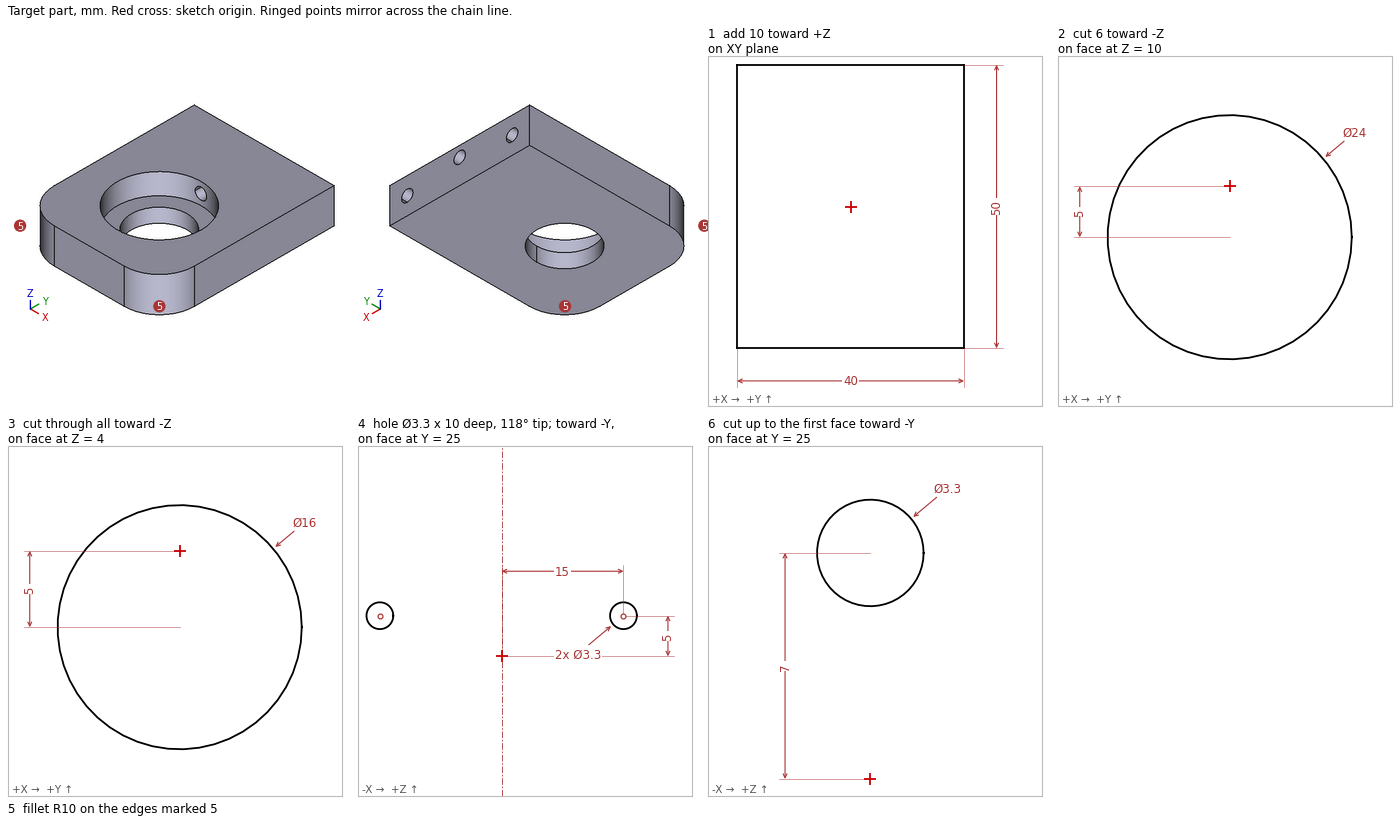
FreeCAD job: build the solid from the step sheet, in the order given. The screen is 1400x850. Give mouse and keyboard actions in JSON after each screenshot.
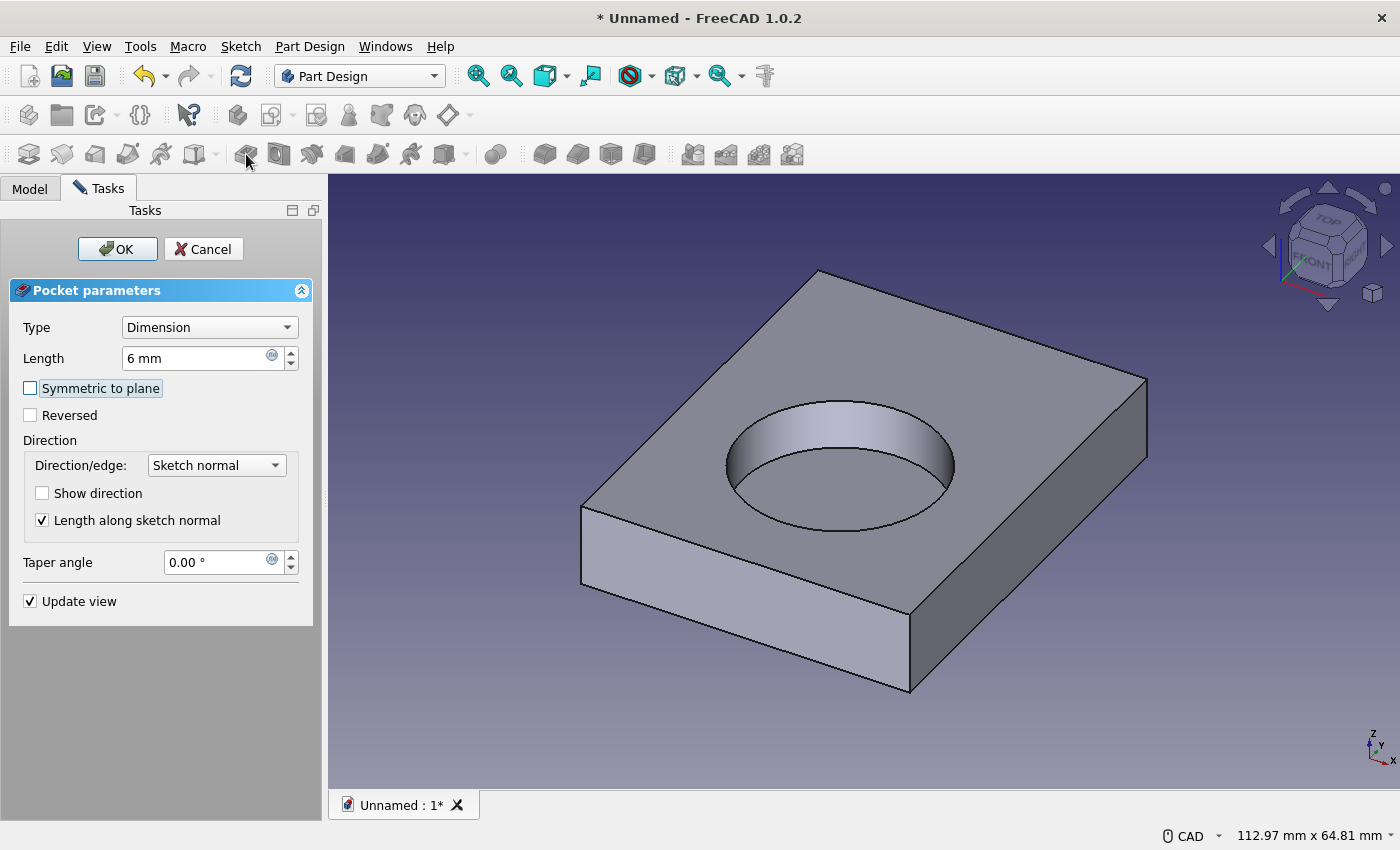
{"action": "left_click", "coordinate": [118, 249]}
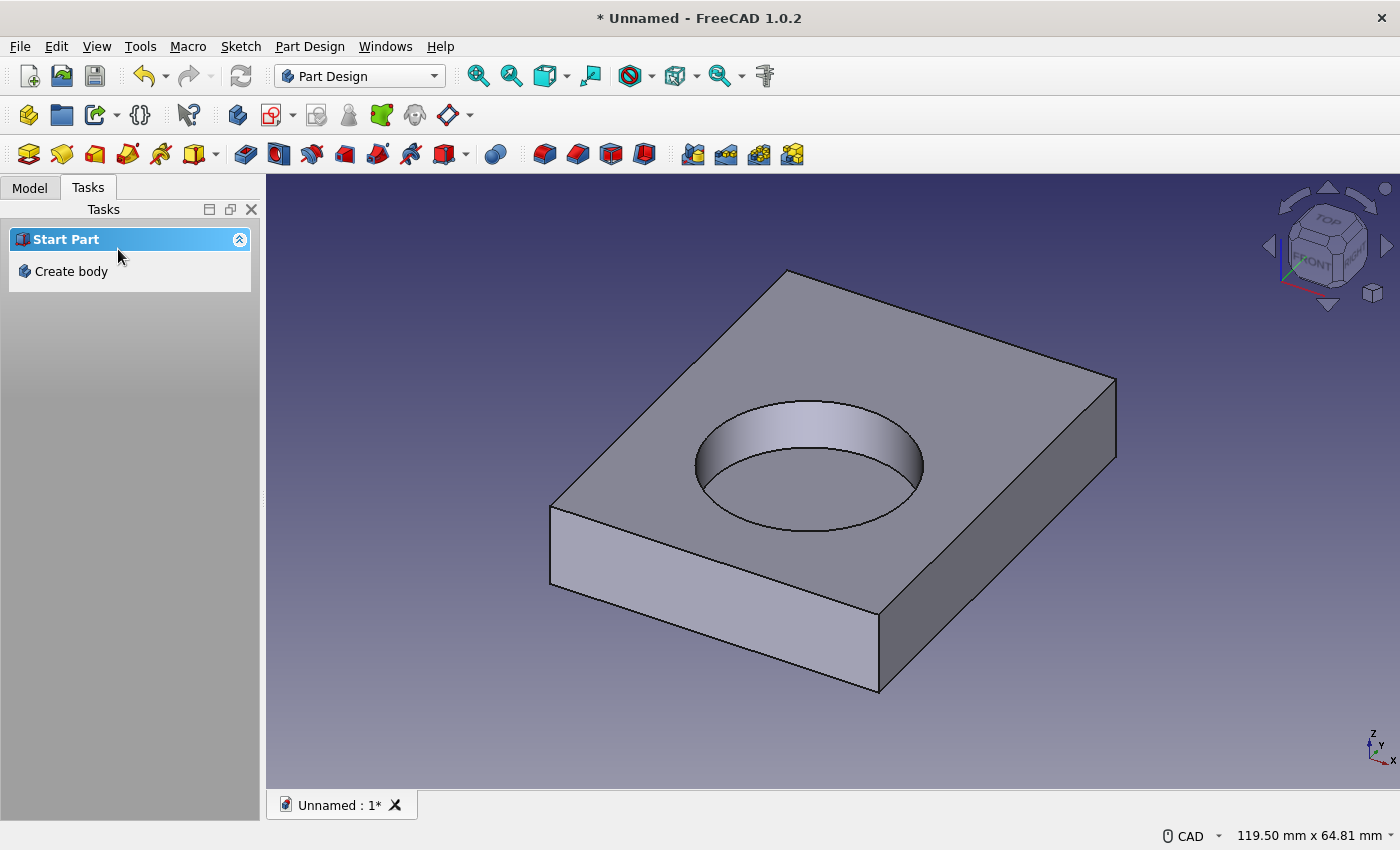
{"action": "left_click", "coordinate": [809, 512]}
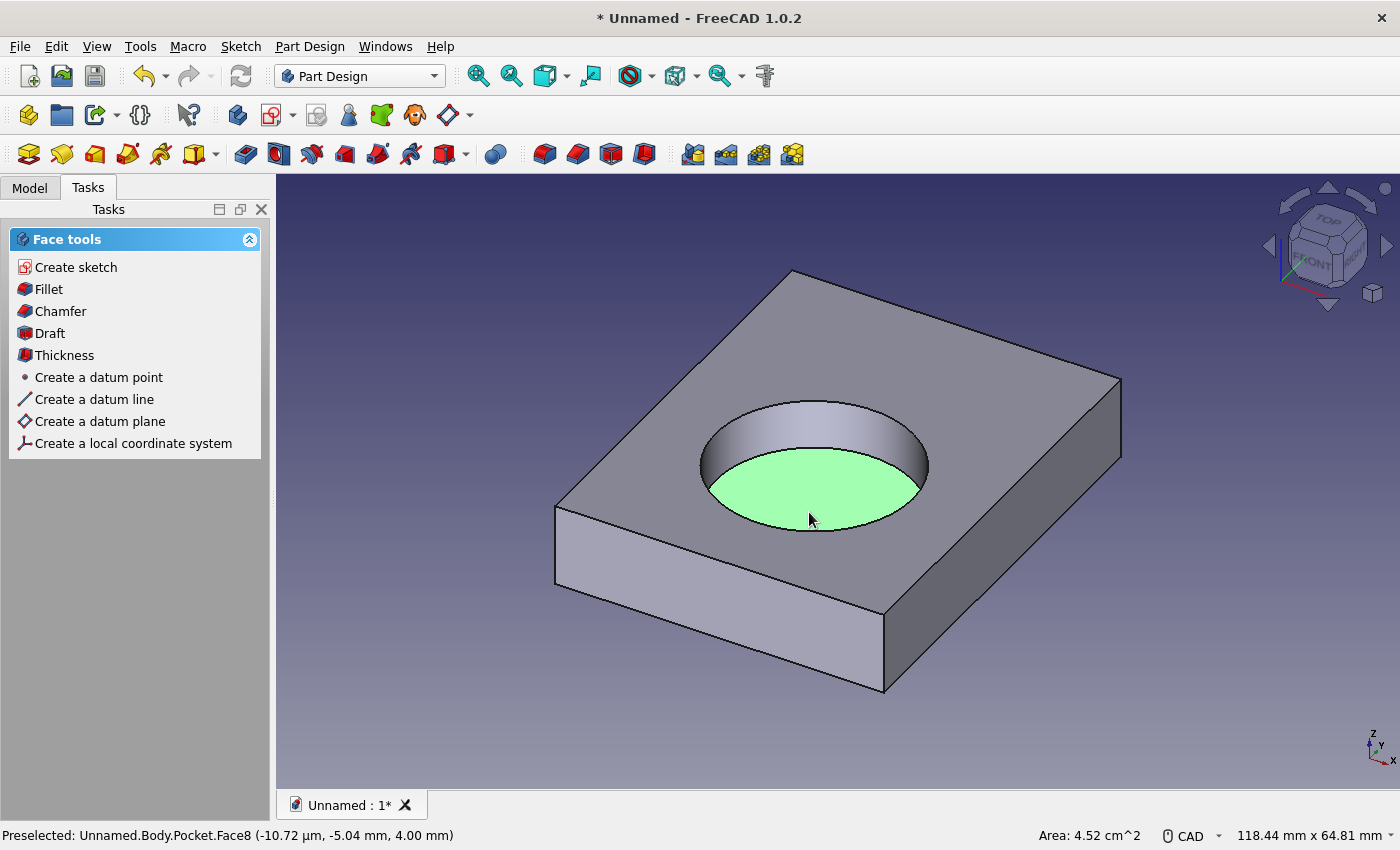
{"action": "left_click", "coordinate": [270, 116]}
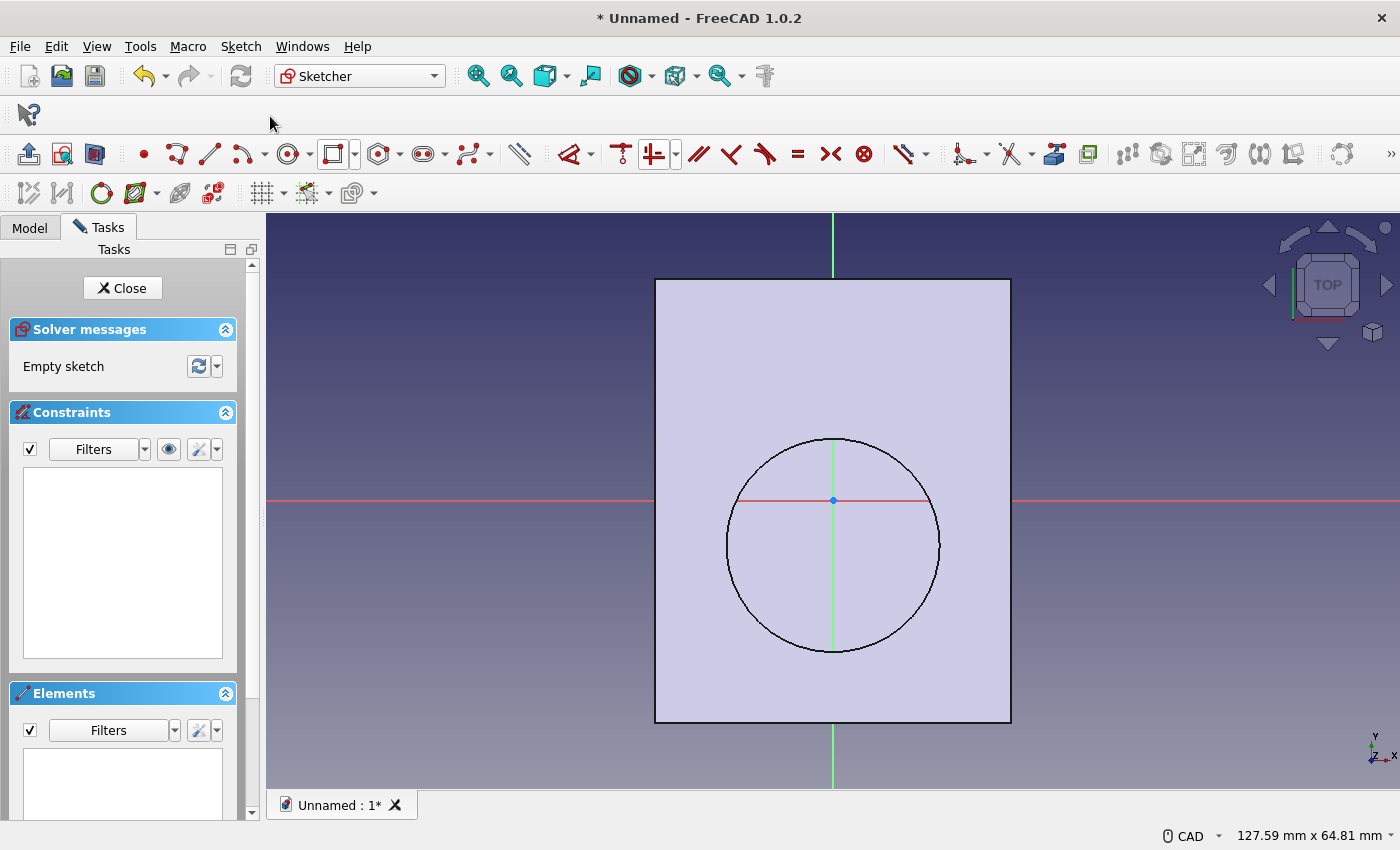
{"action": "left_click", "coordinate": [95, 154]}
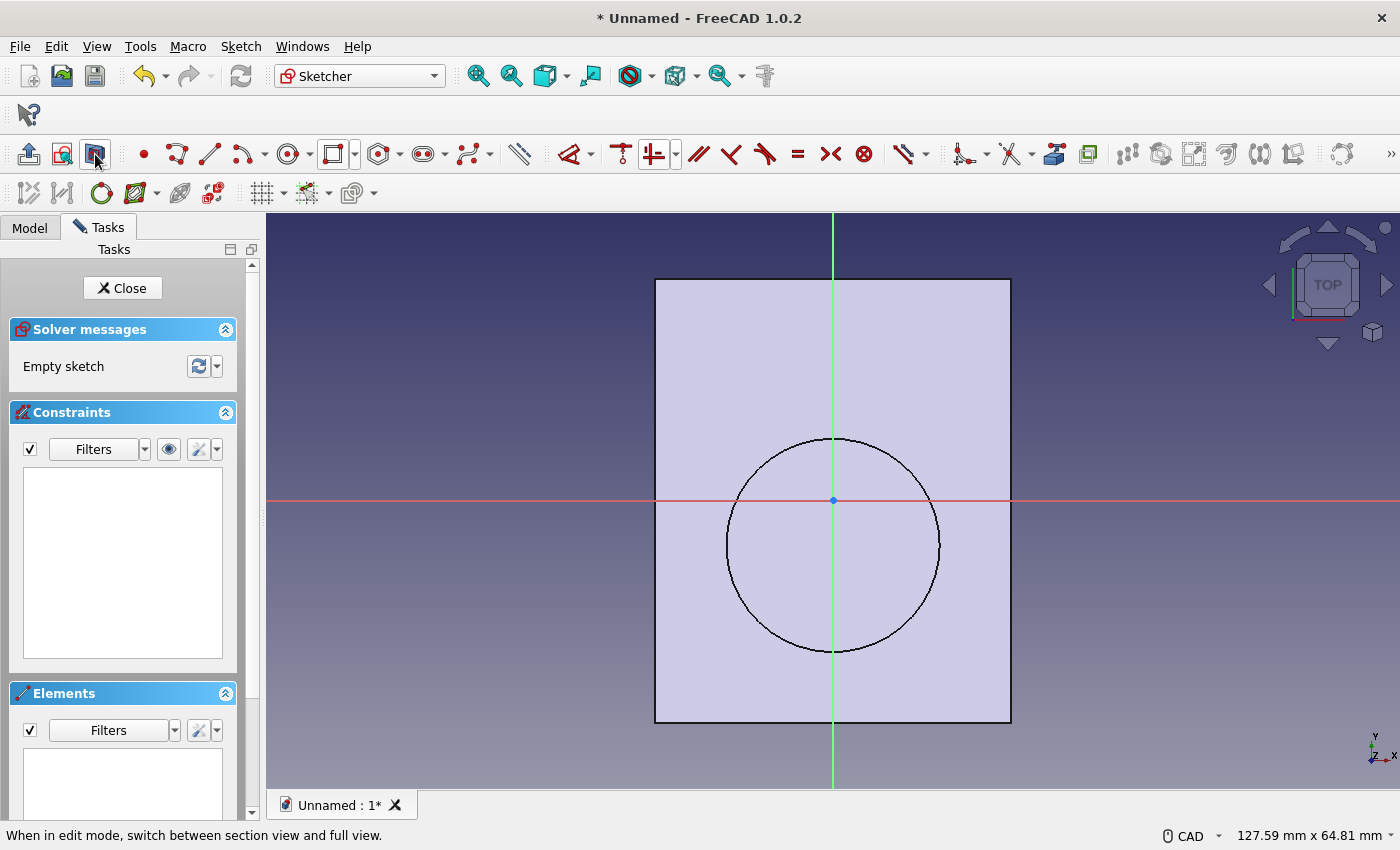
{"action": "scroll", "coordinate": [873, 571], "scroll_direction": "up", "scroll_amount": 5}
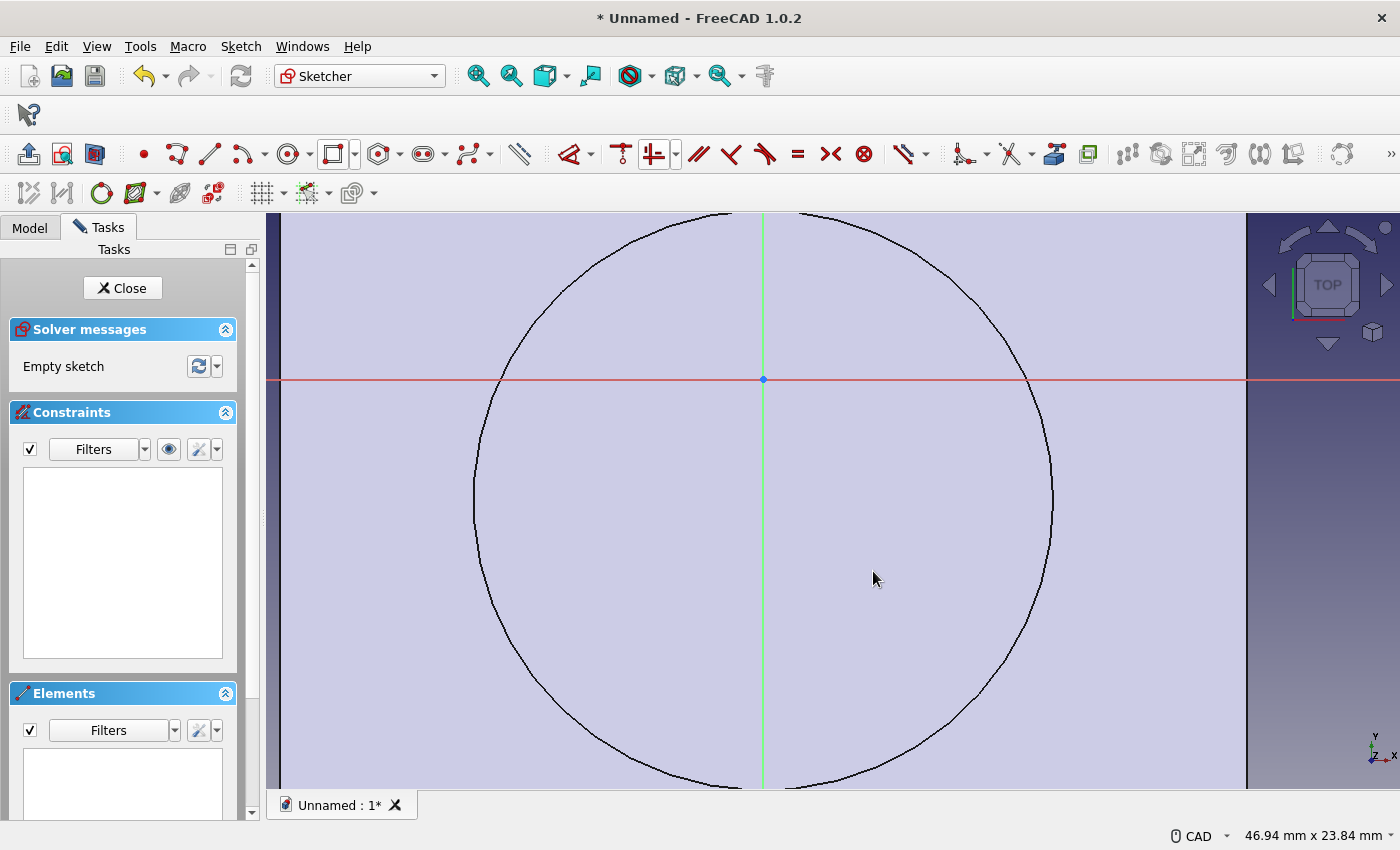
{"action": "left_click", "coordinate": [288, 154]}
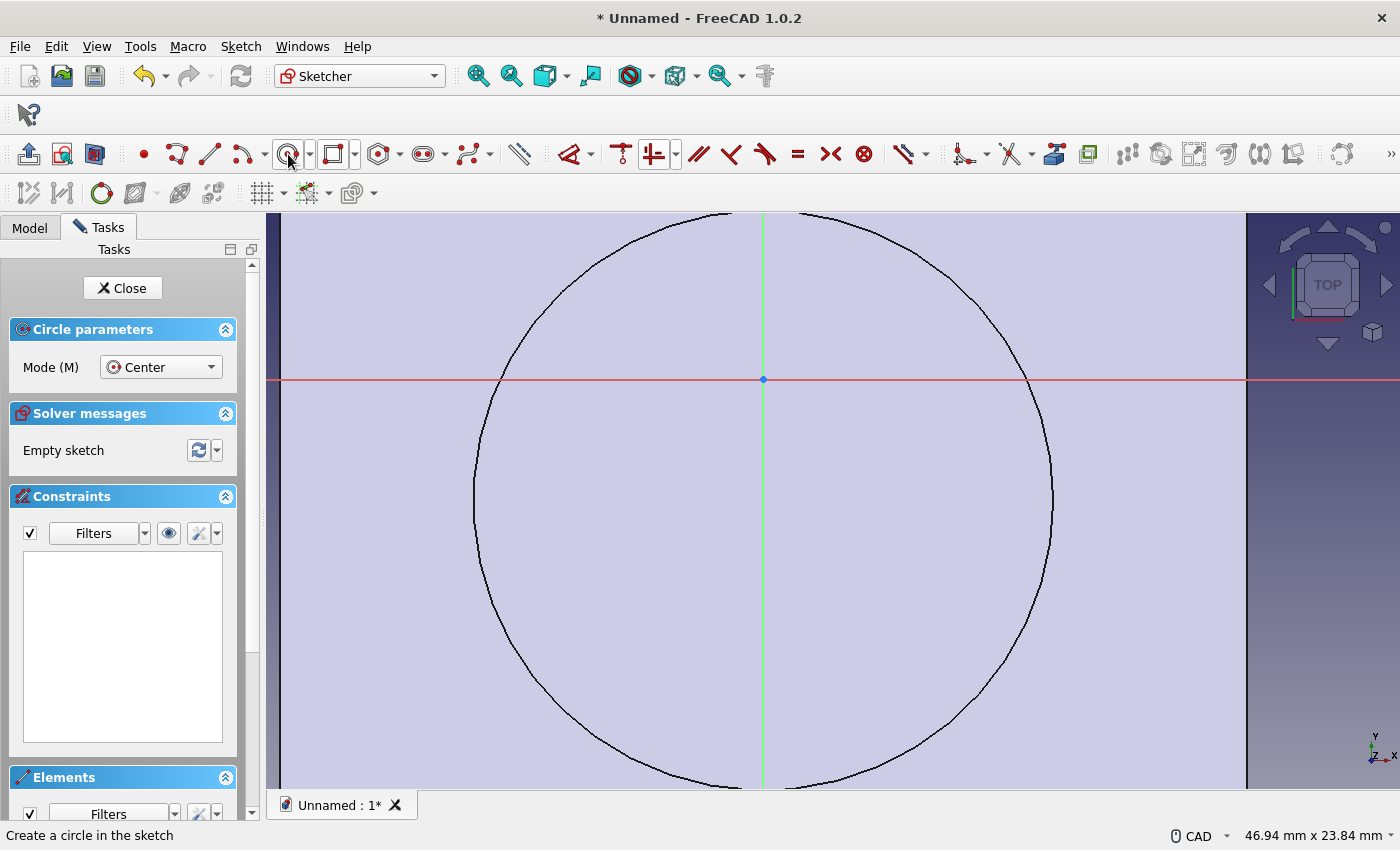
{"action": "left_click", "coordinate": [763, 500]}
{"action": "mouse_move", "coordinate": [900, 364]}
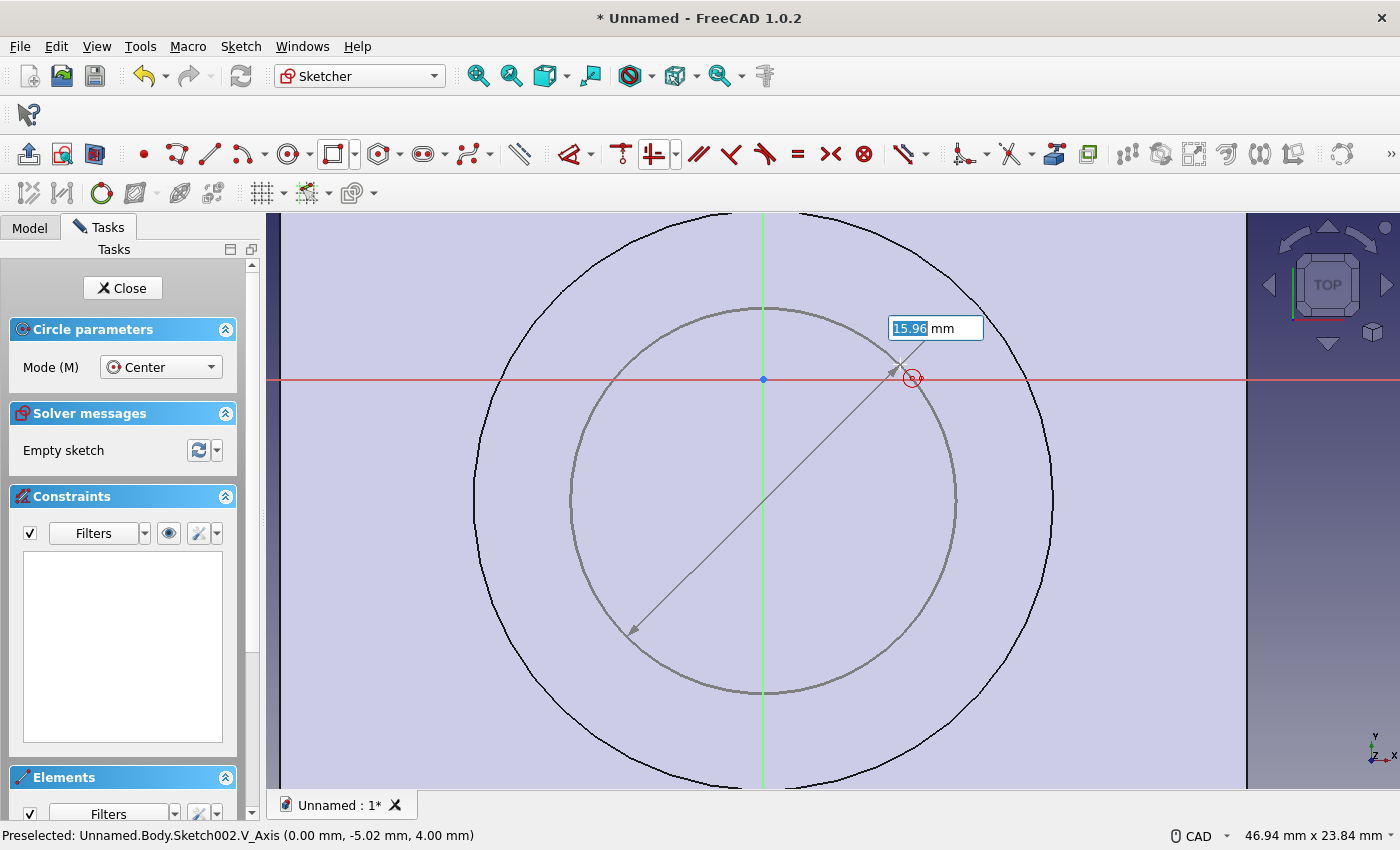
{"action": "type", "text": "16"}
{"action": "key", "text": "Return"}
{"action": "key", "text": "Escape"}